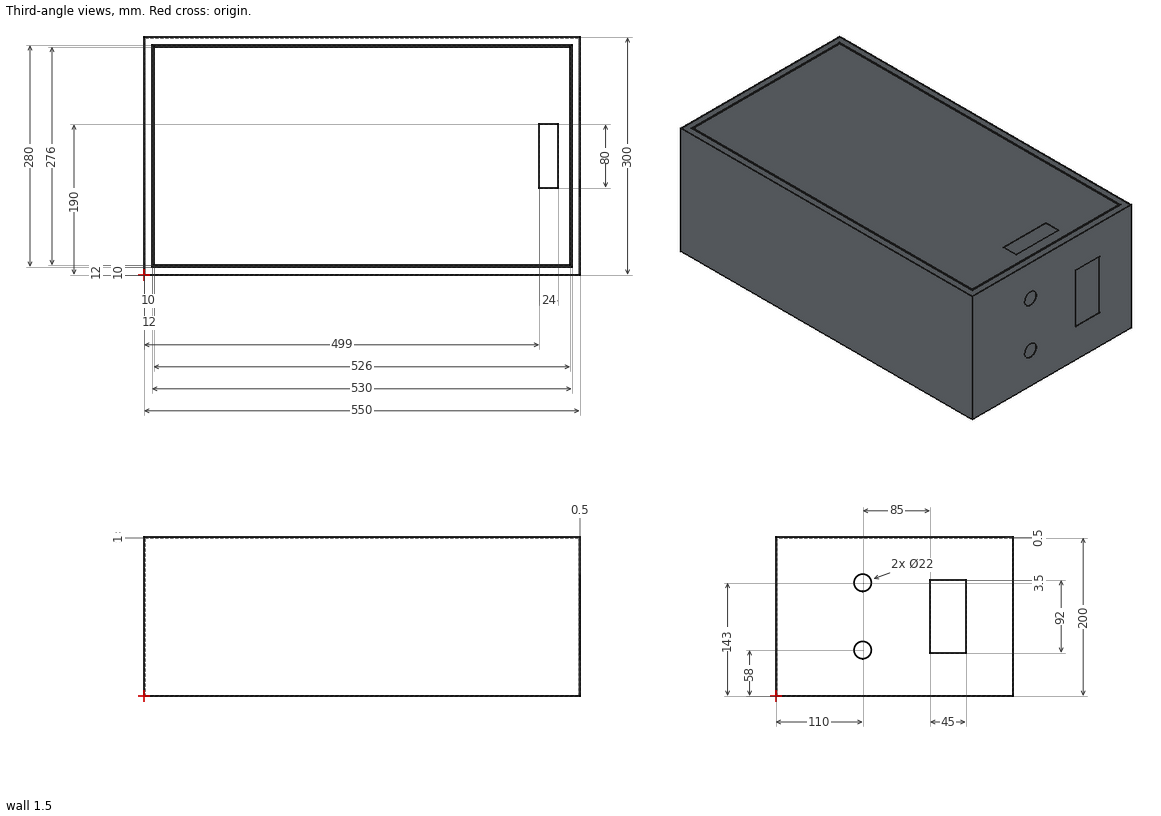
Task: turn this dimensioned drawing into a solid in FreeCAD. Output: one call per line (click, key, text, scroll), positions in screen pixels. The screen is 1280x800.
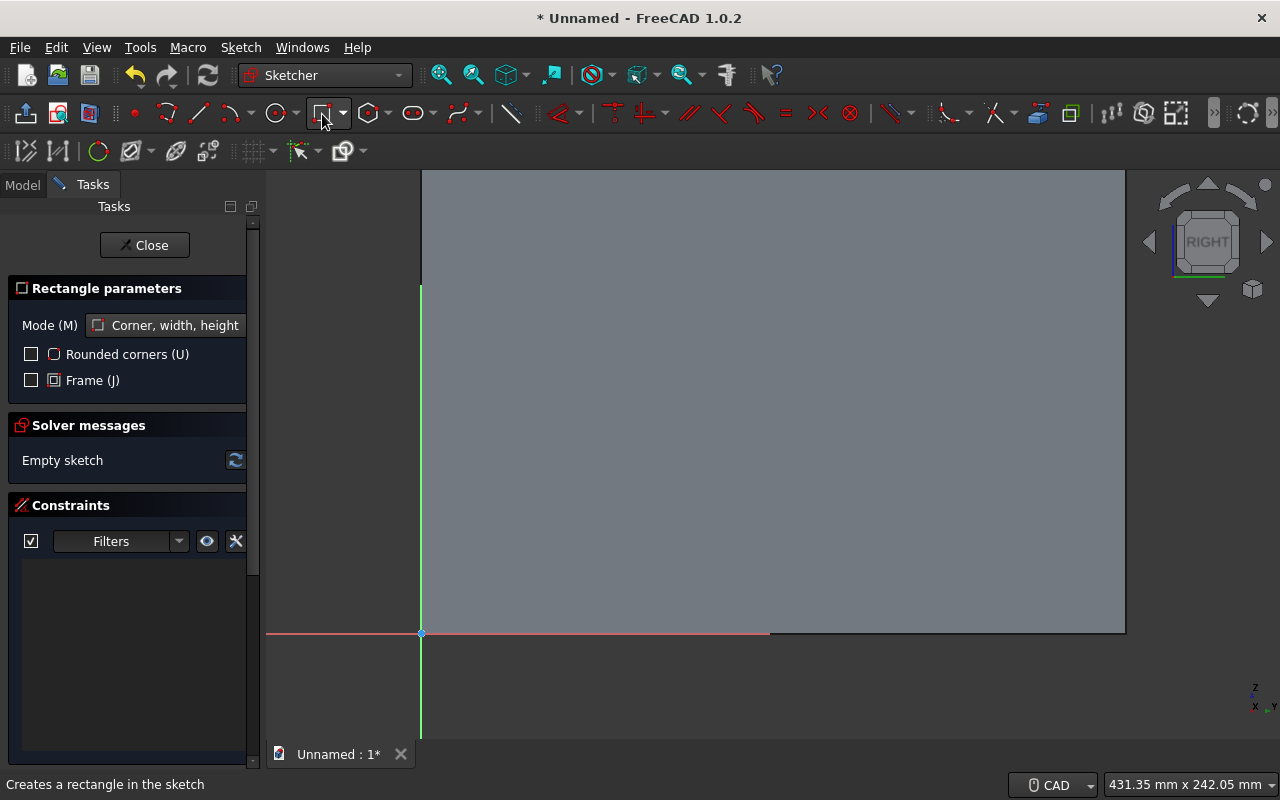
click(880, 290)
move(985, 506)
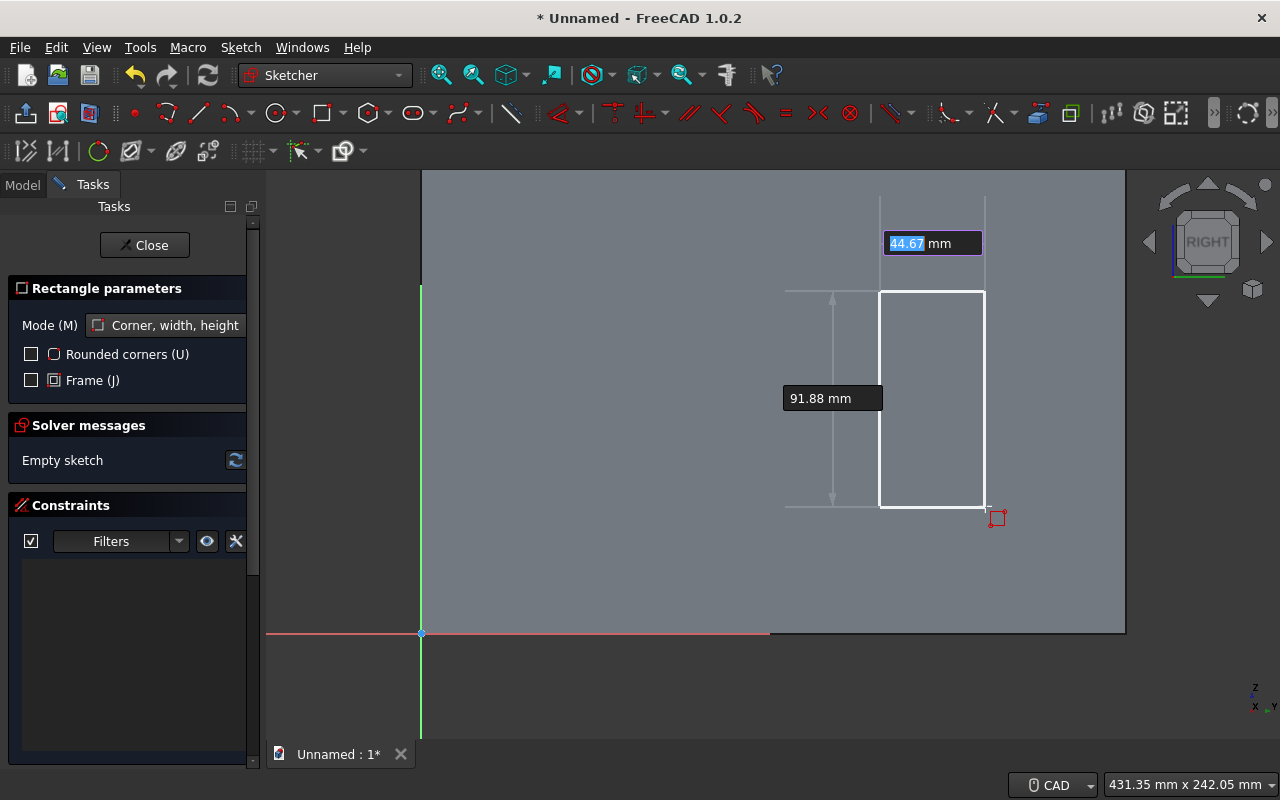
text(45)
key(Tab)
text(92)
key(Return)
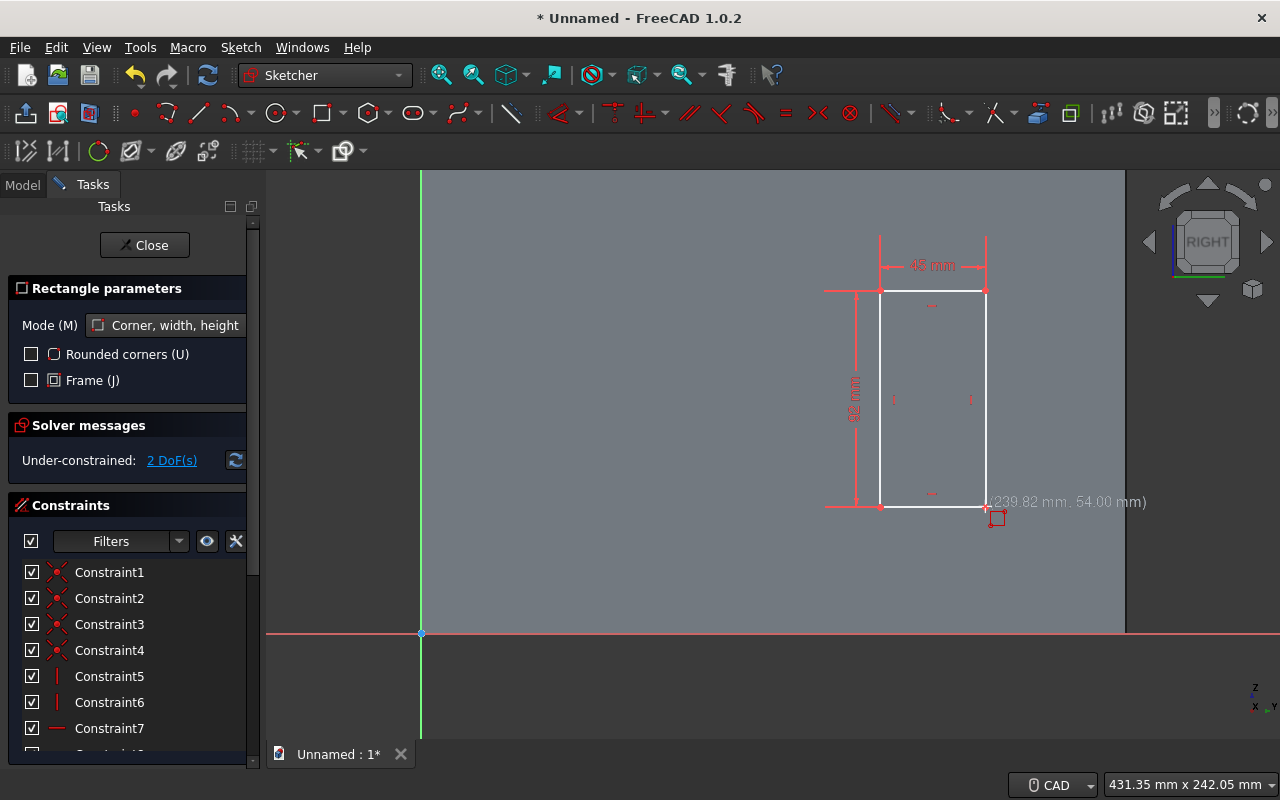
click(276, 114)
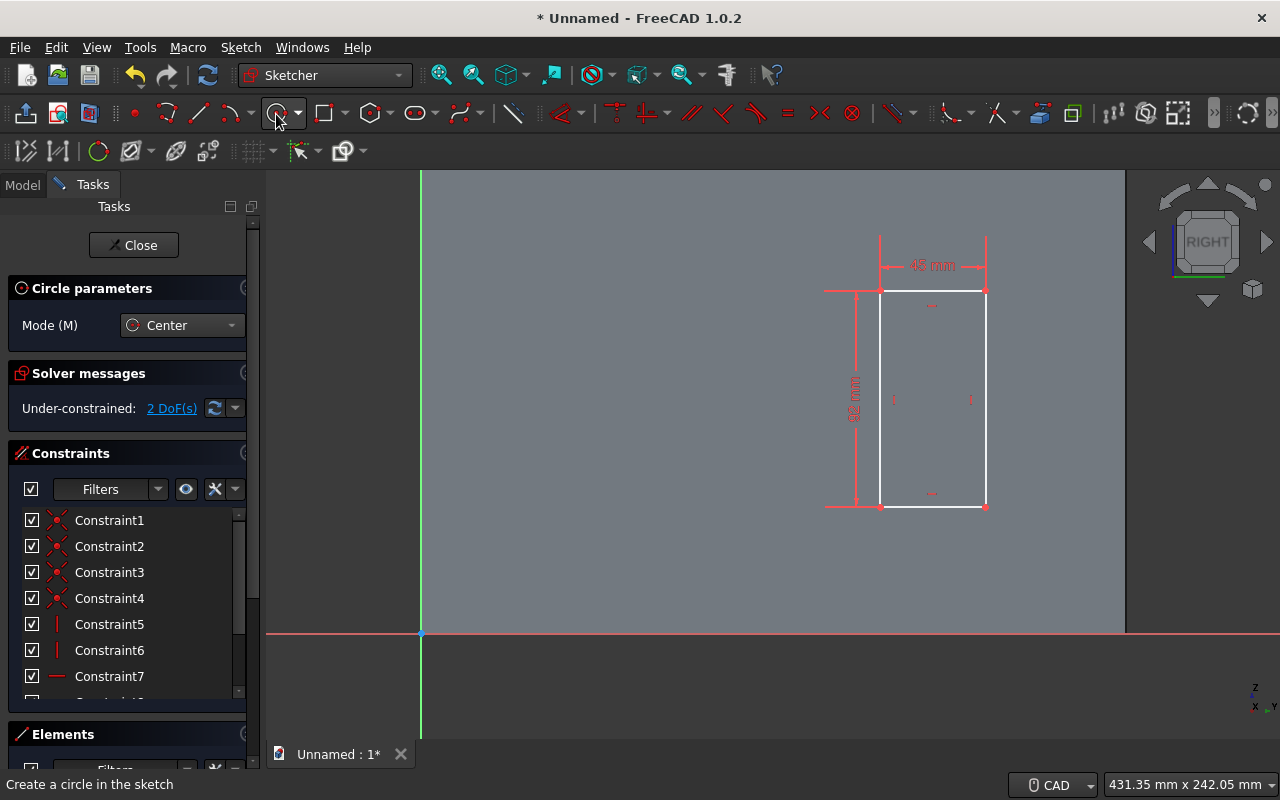
click(680, 298)
move(698, 280)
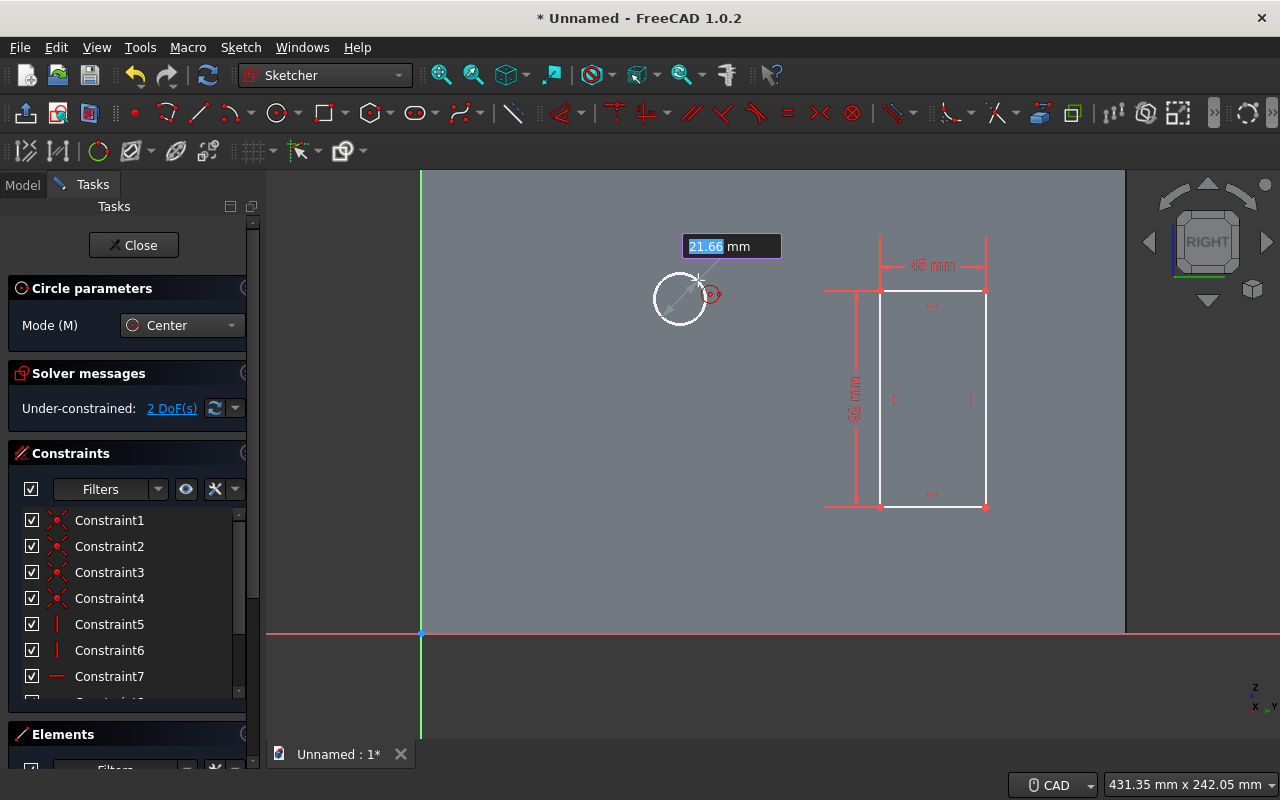
text(22)
key(Return)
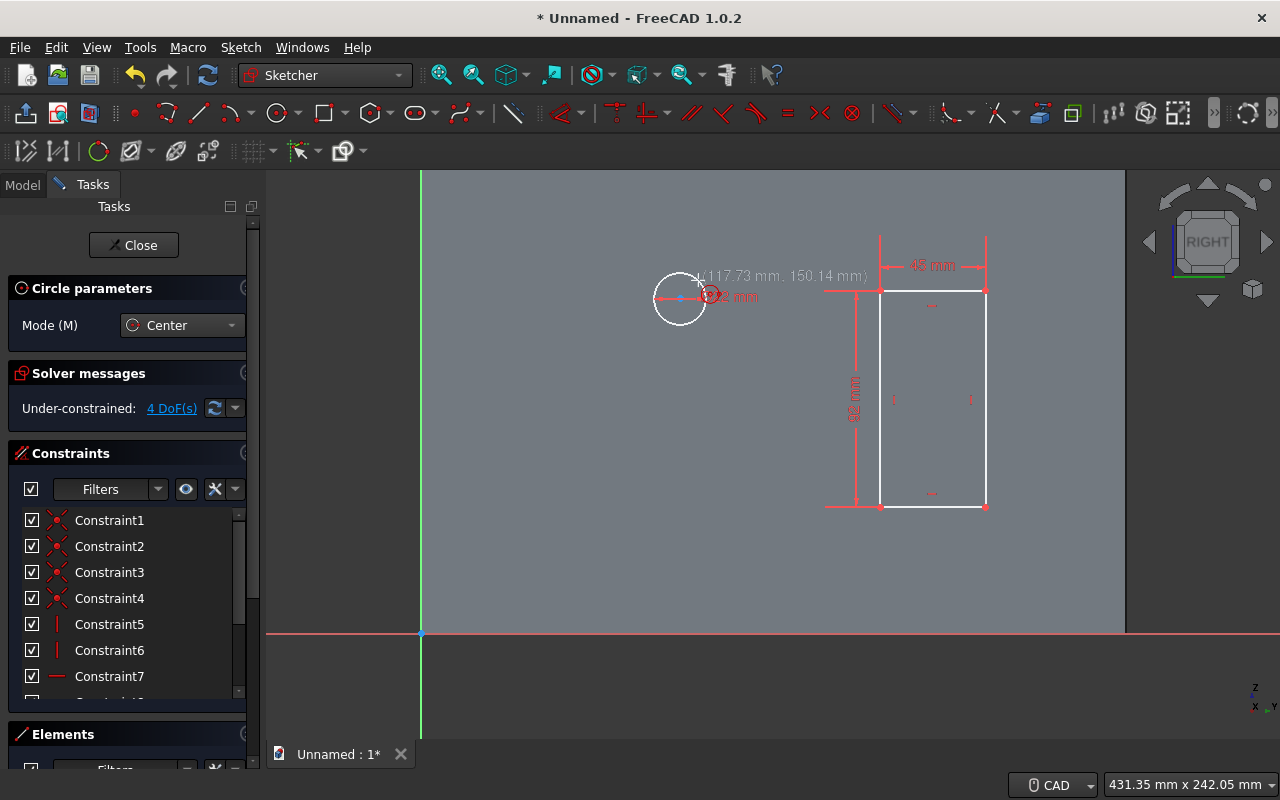
click(680, 498)
move(698, 479)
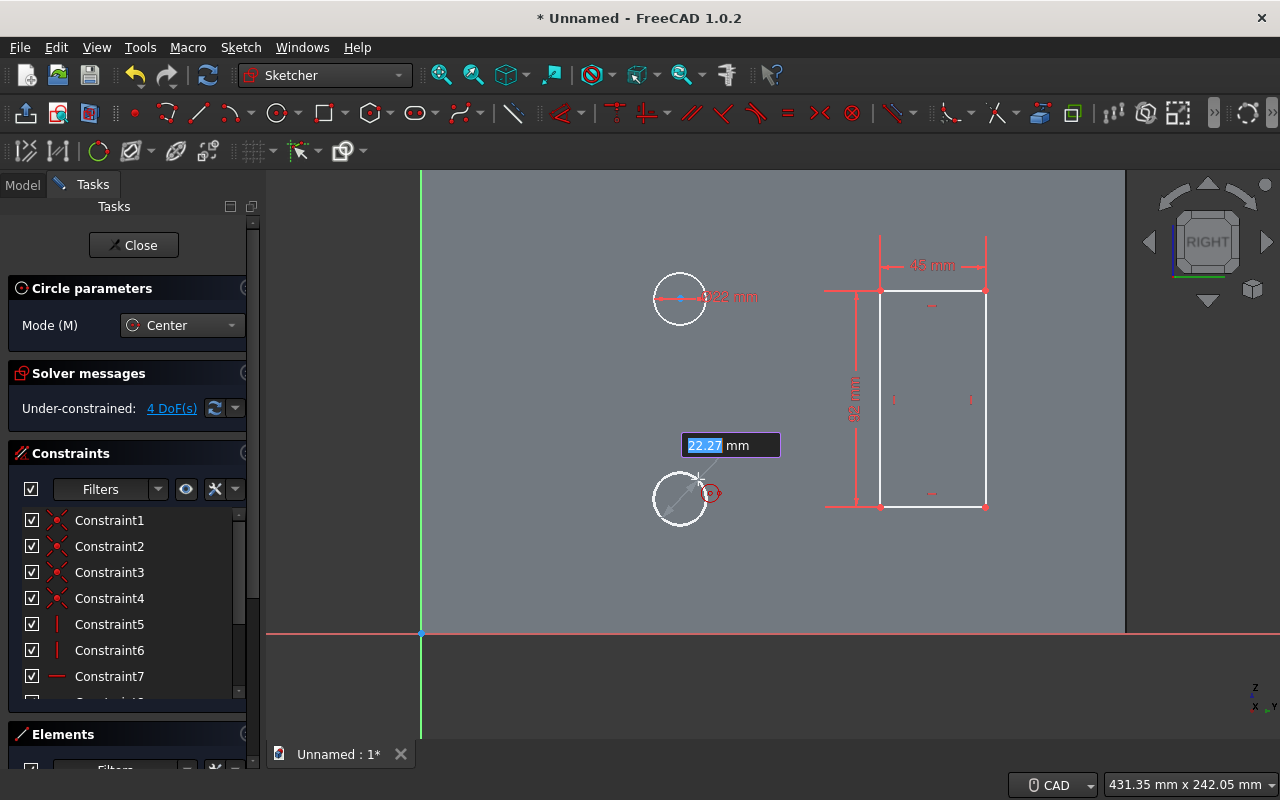
text(22)
key(Return)
key(Escape)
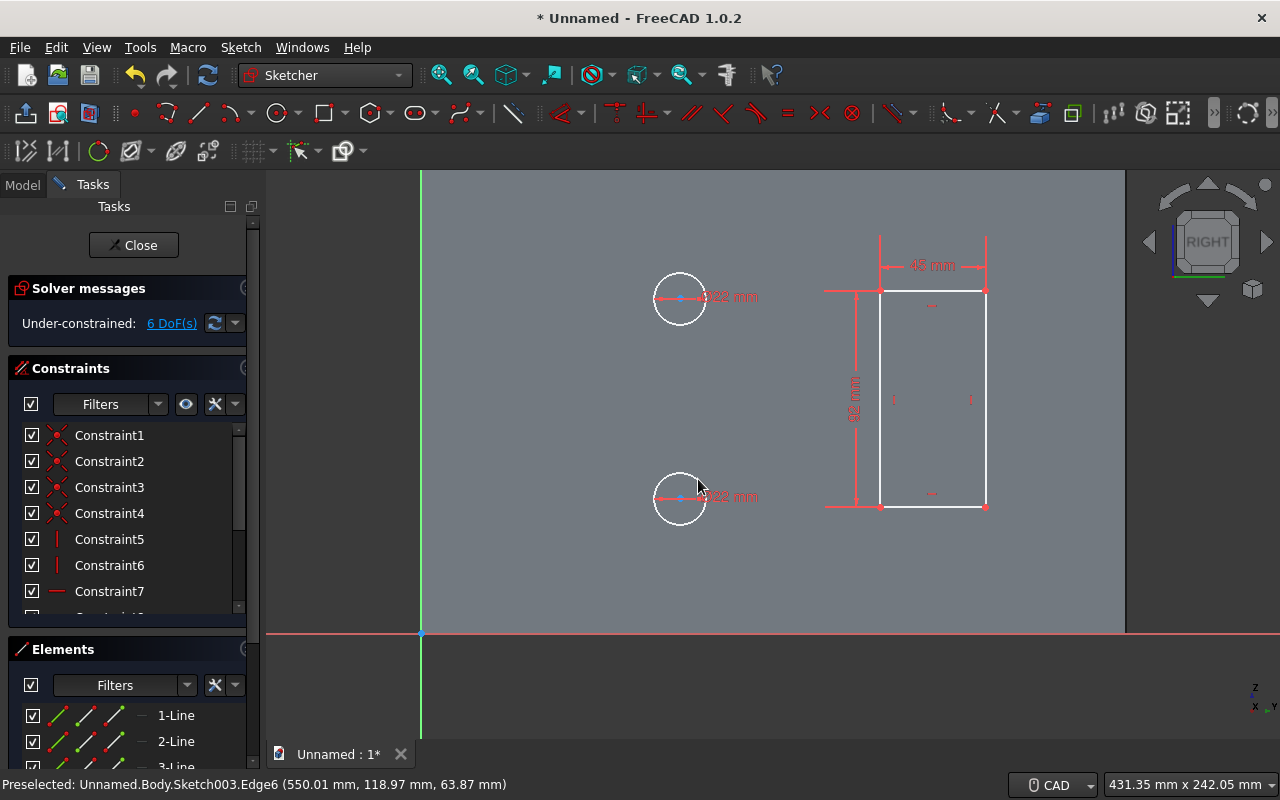
click(680, 299)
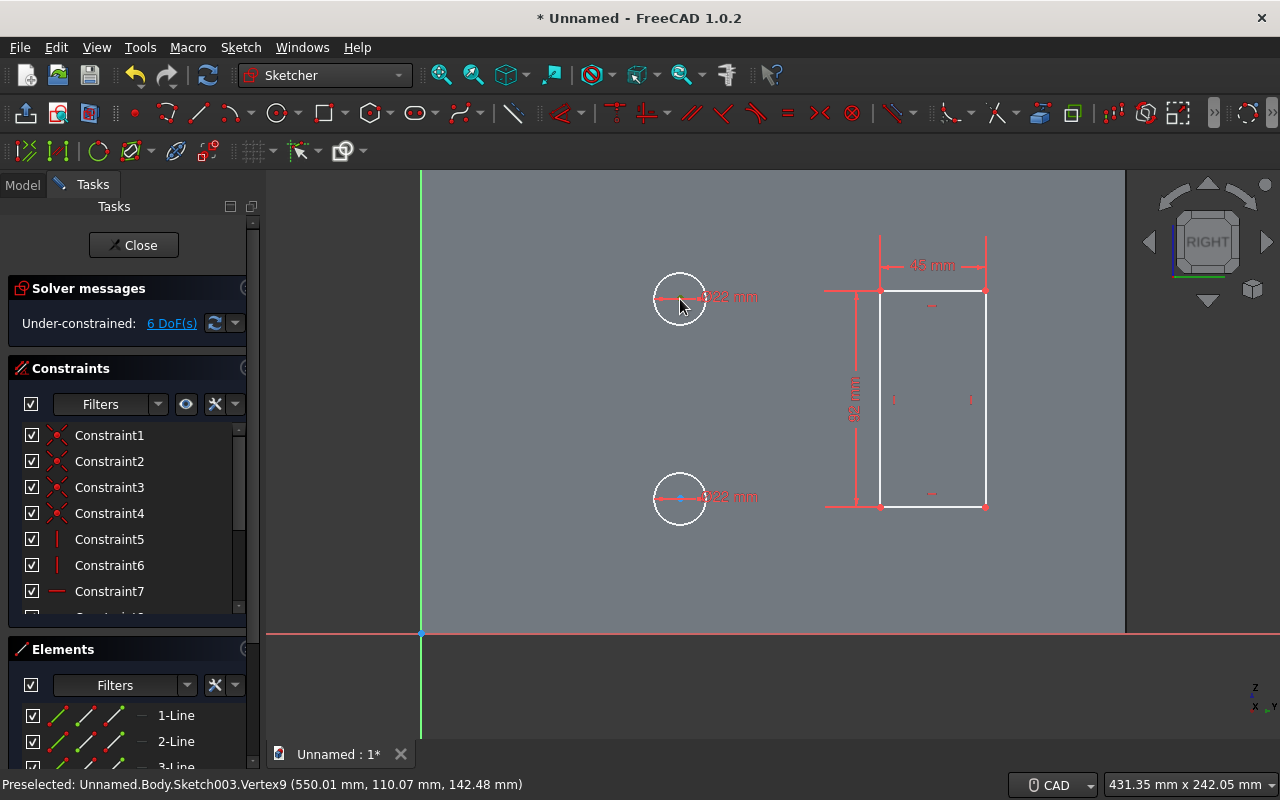
click(680, 499)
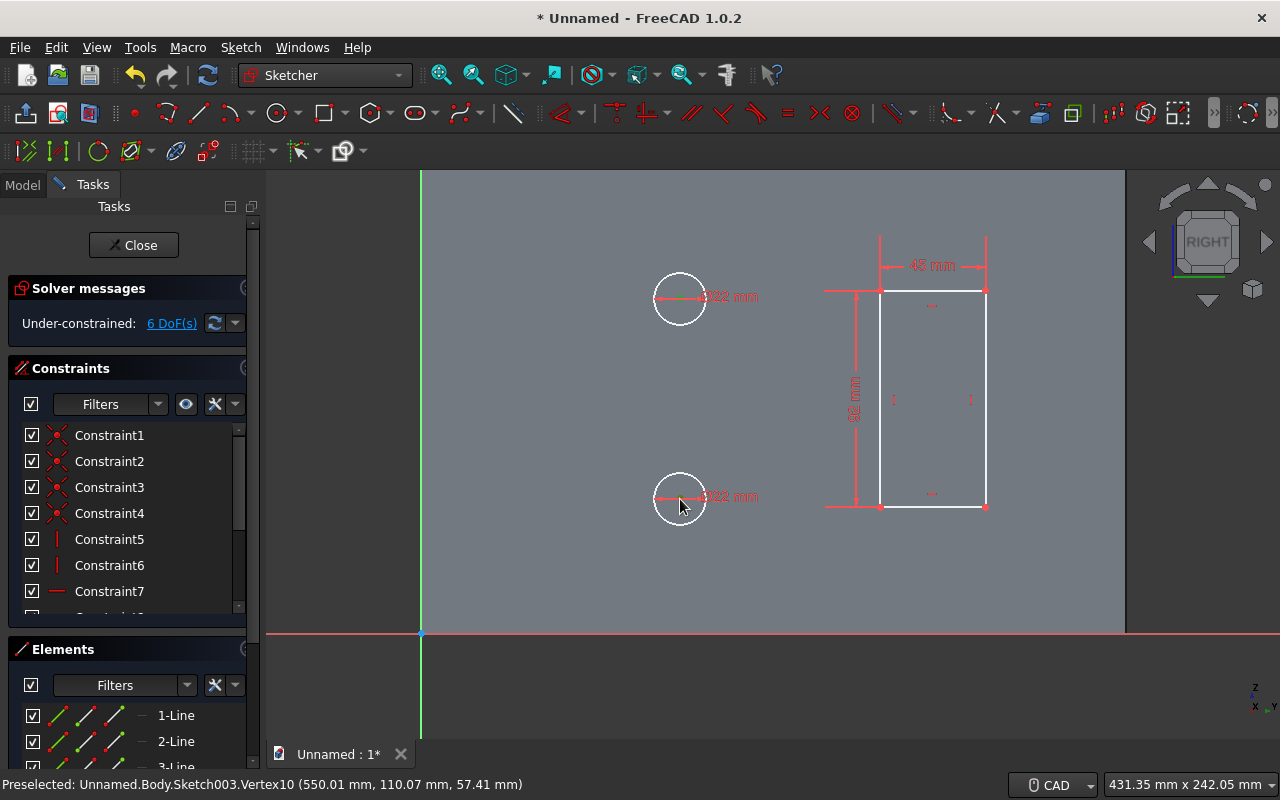
click(670, 114)